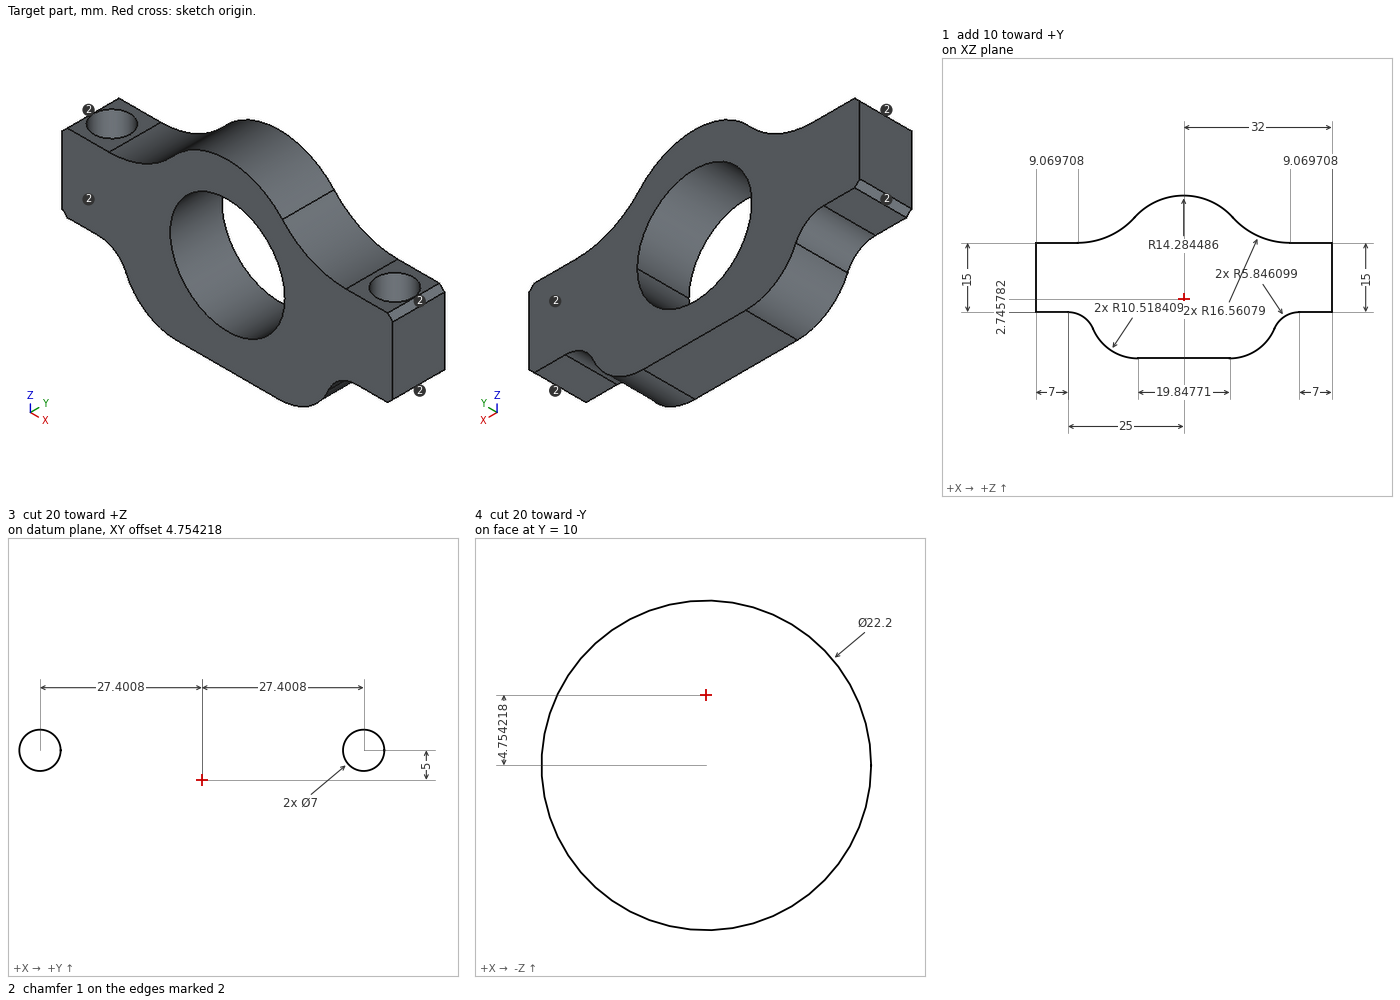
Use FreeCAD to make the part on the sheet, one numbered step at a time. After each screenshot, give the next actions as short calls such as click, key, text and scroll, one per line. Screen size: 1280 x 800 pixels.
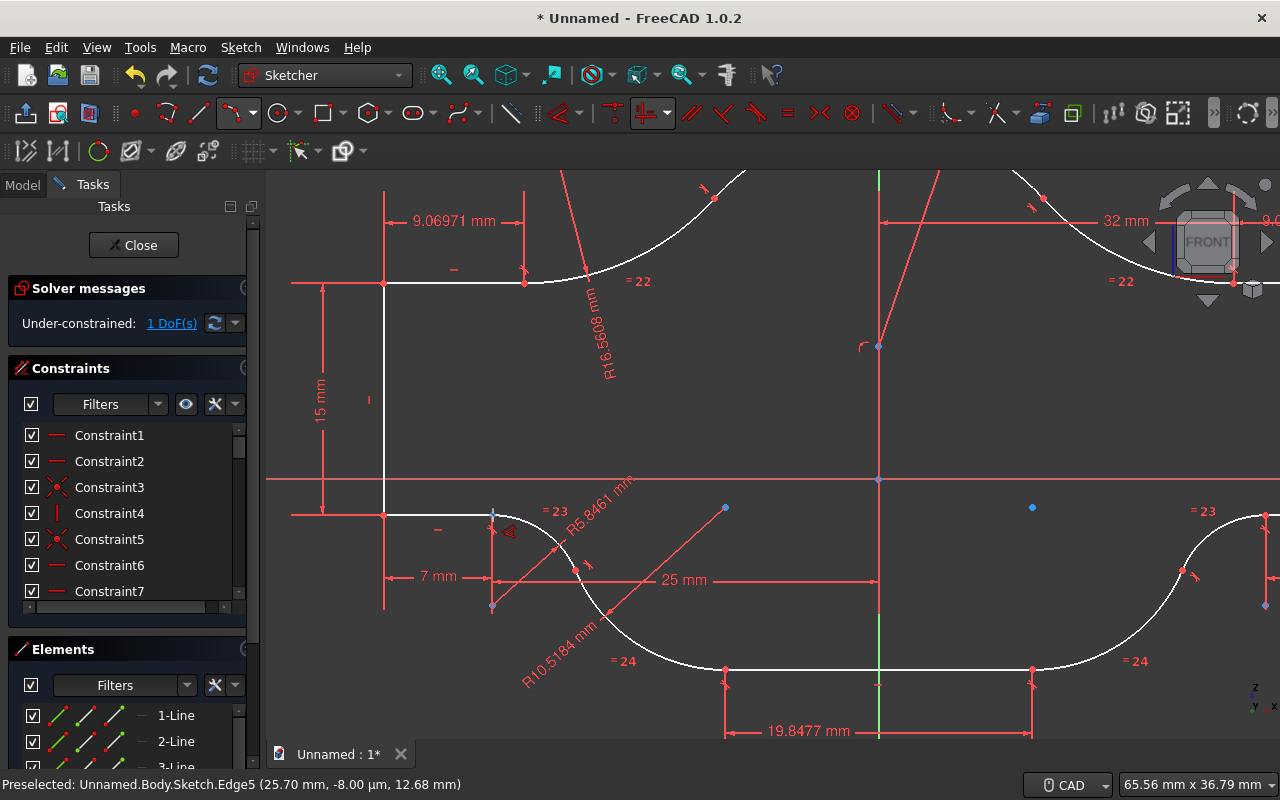
click(492, 515)
click(458, 497)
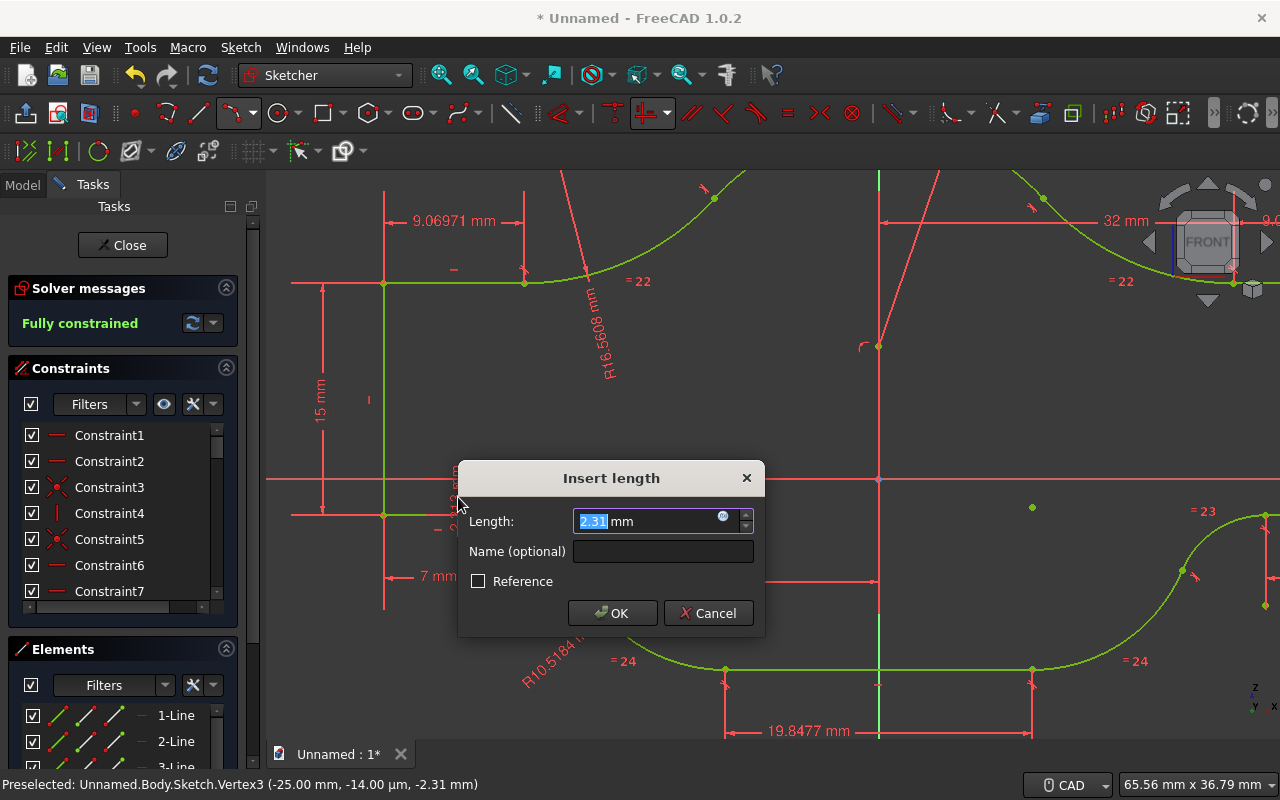
text(2.745782)
key(Return)
key(Escape)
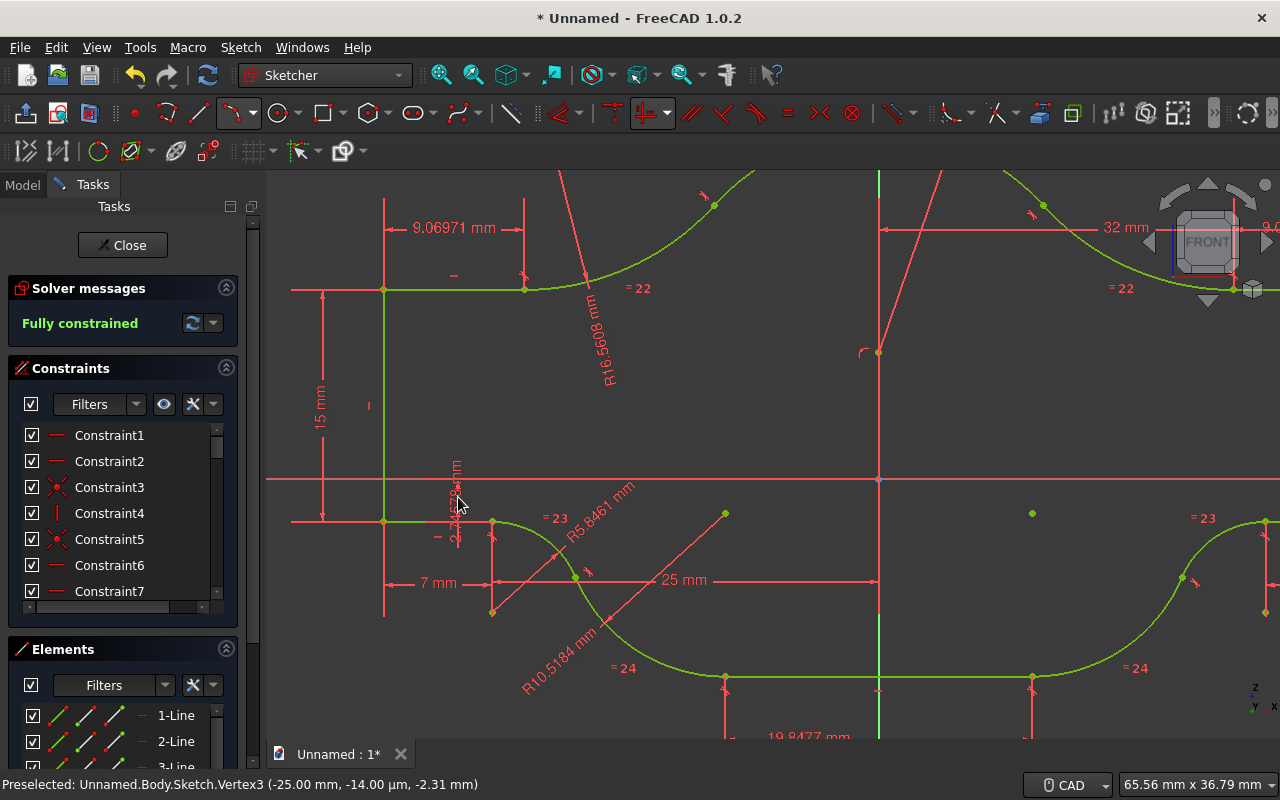
click(123, 245)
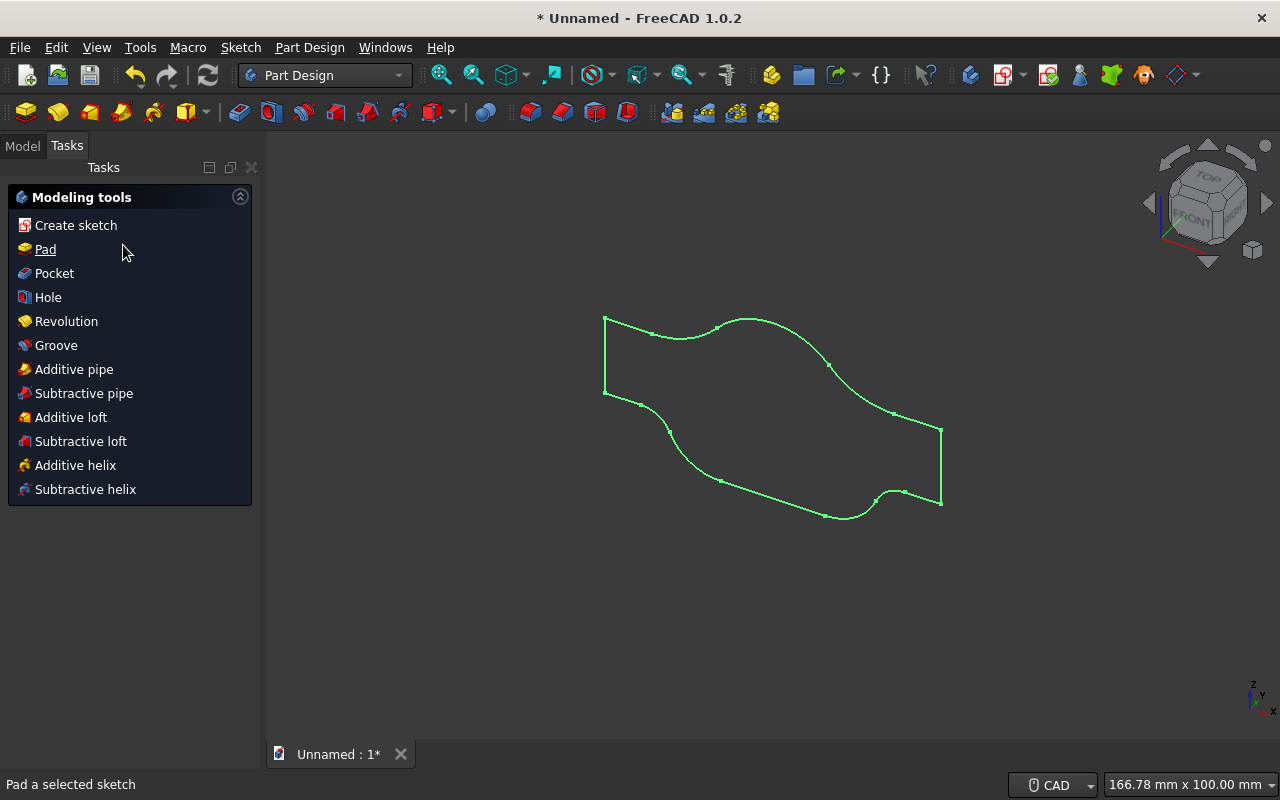
click(26, 112)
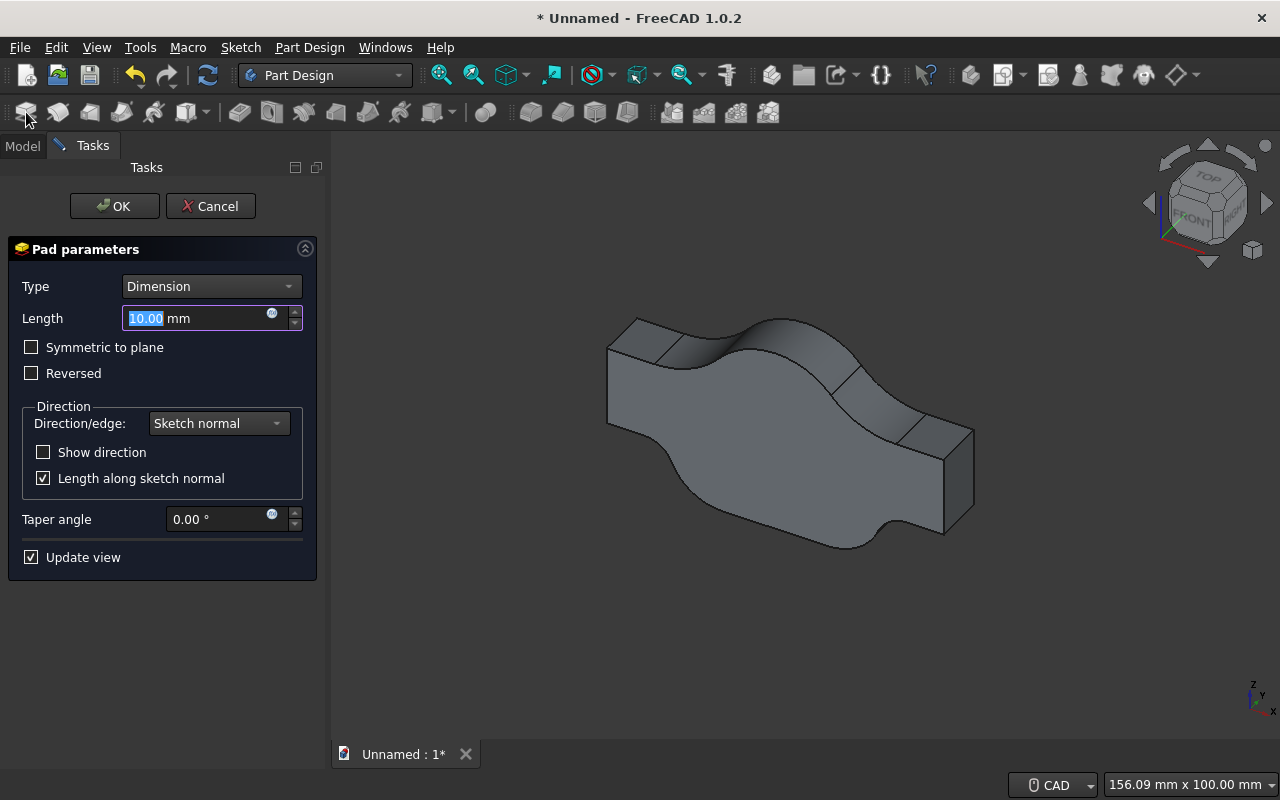
text(10)
key(Tab)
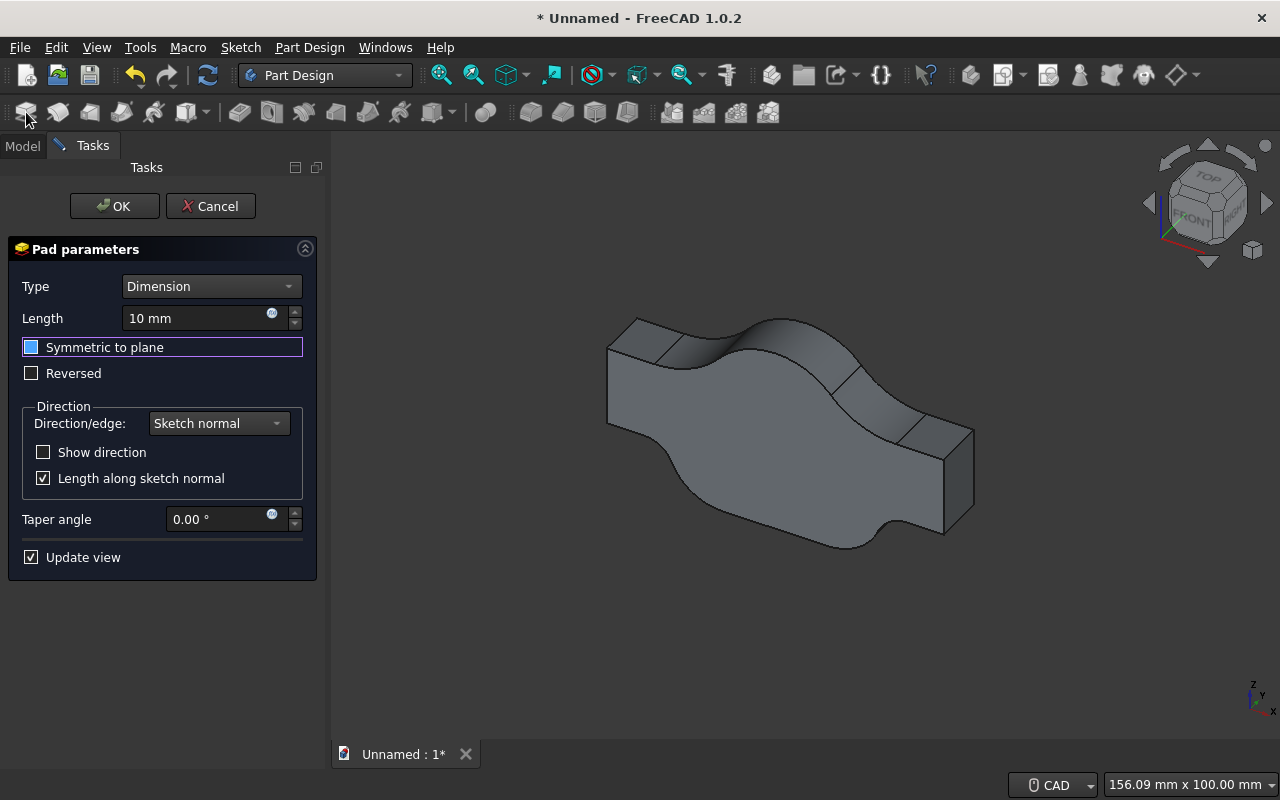
click(30, 373)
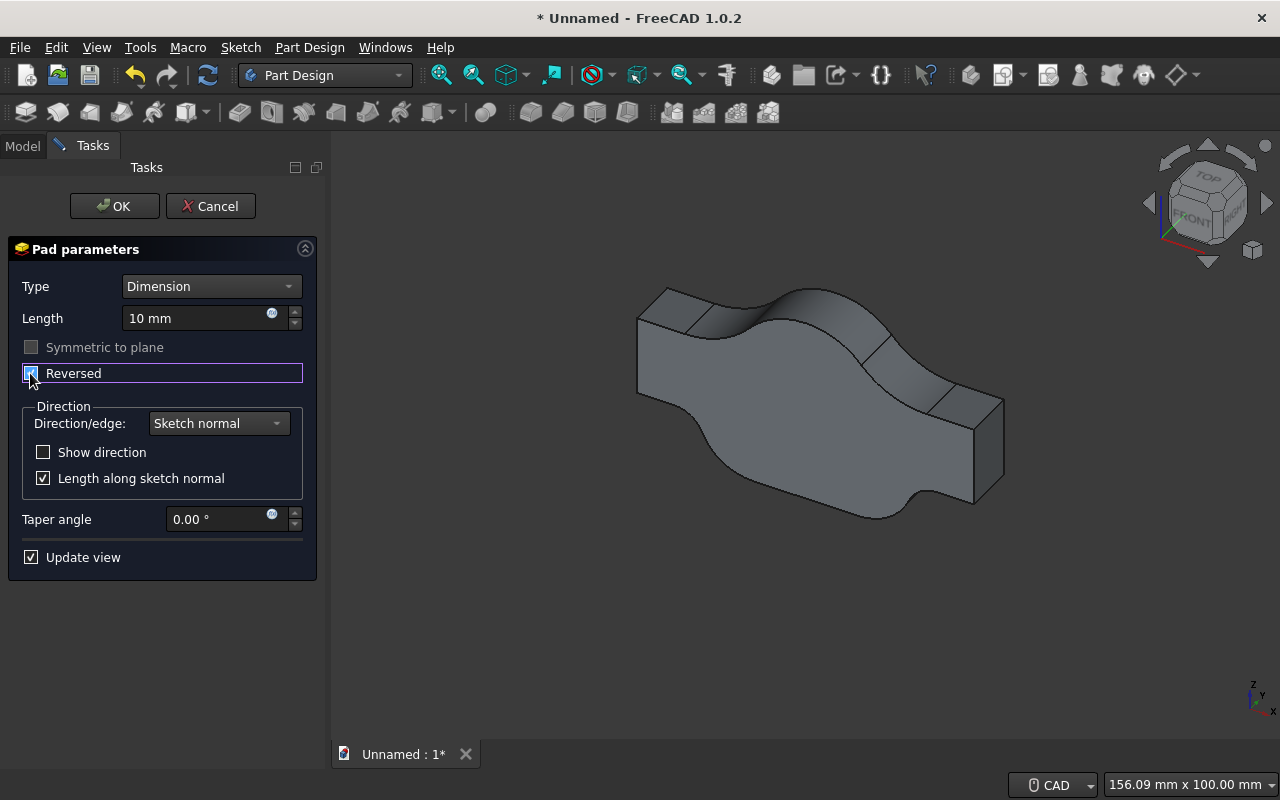
click(115, 206)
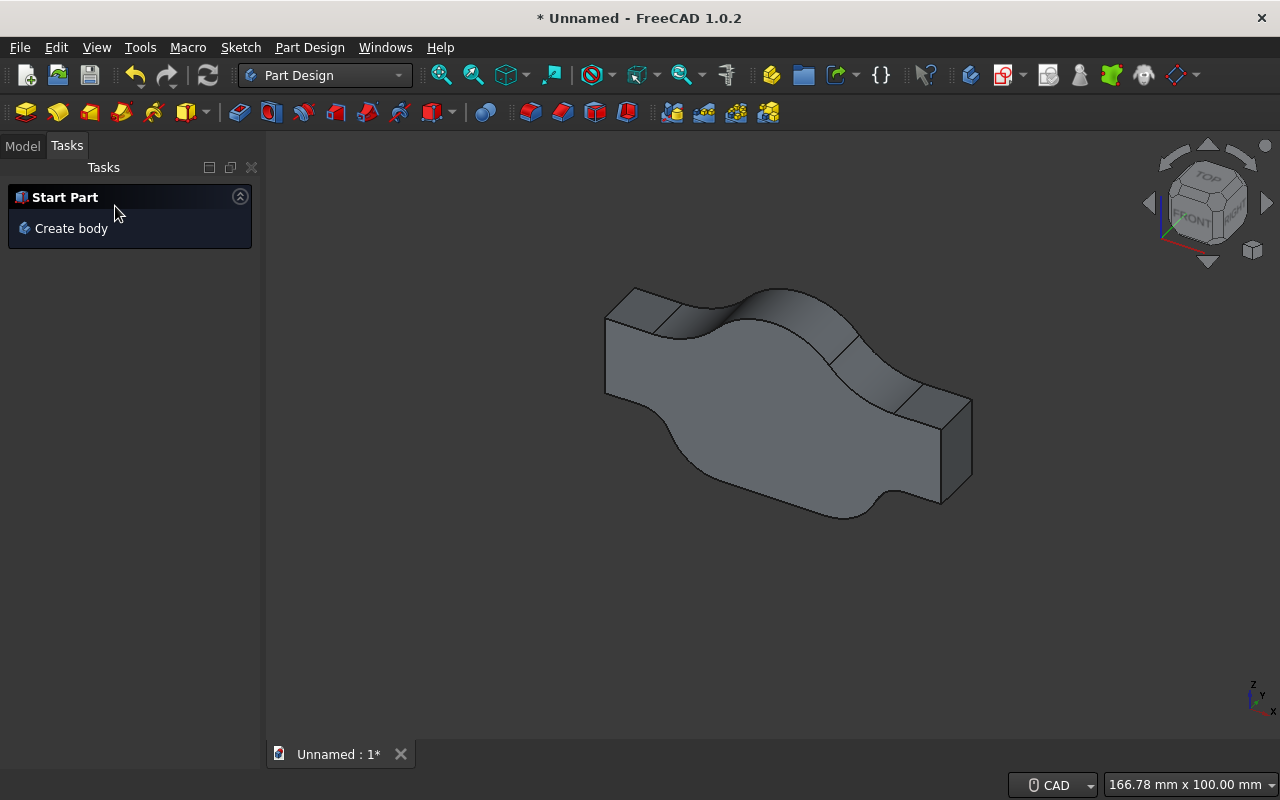
click(957, 414)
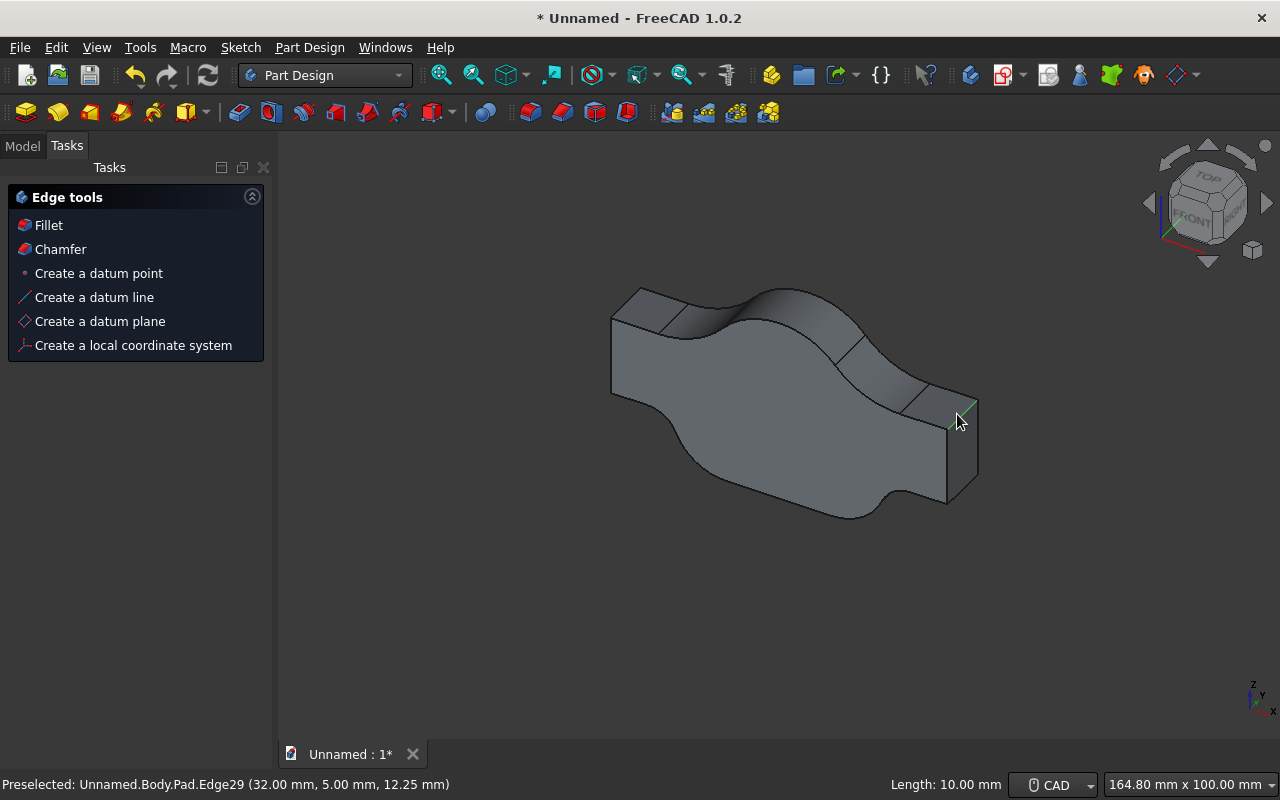
key(0)